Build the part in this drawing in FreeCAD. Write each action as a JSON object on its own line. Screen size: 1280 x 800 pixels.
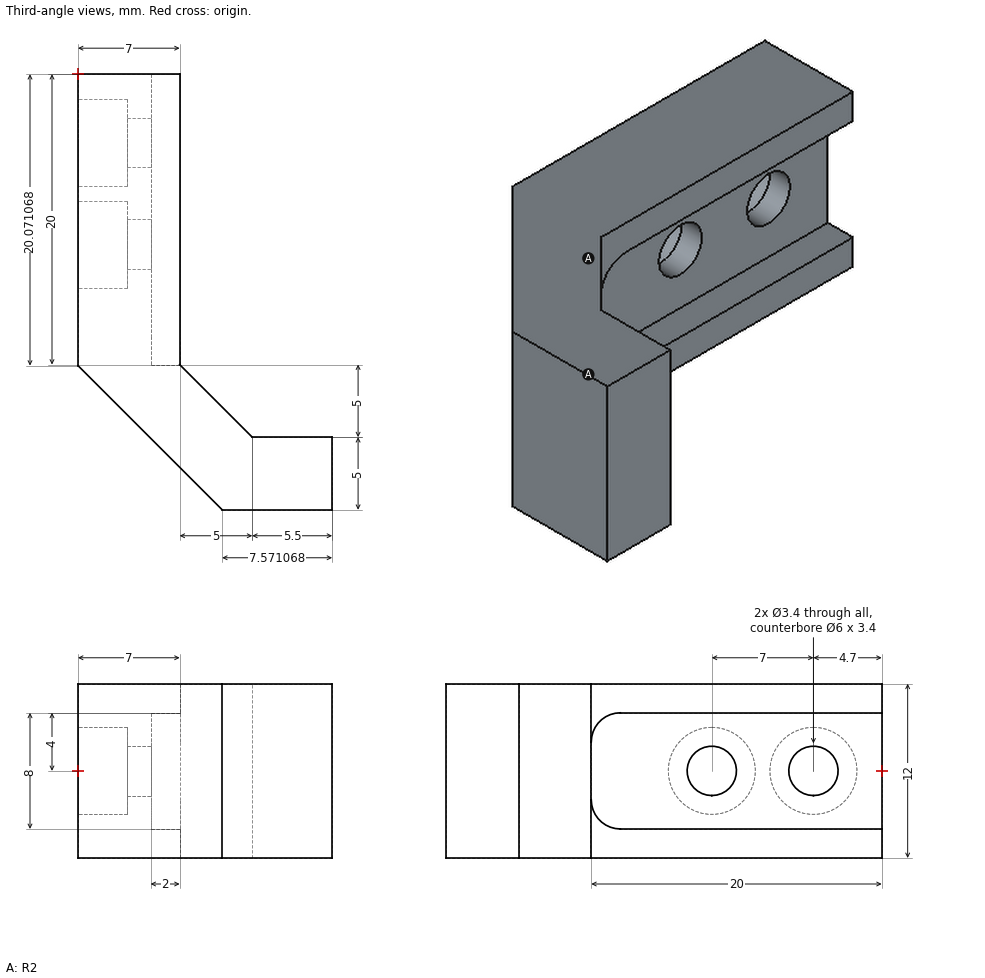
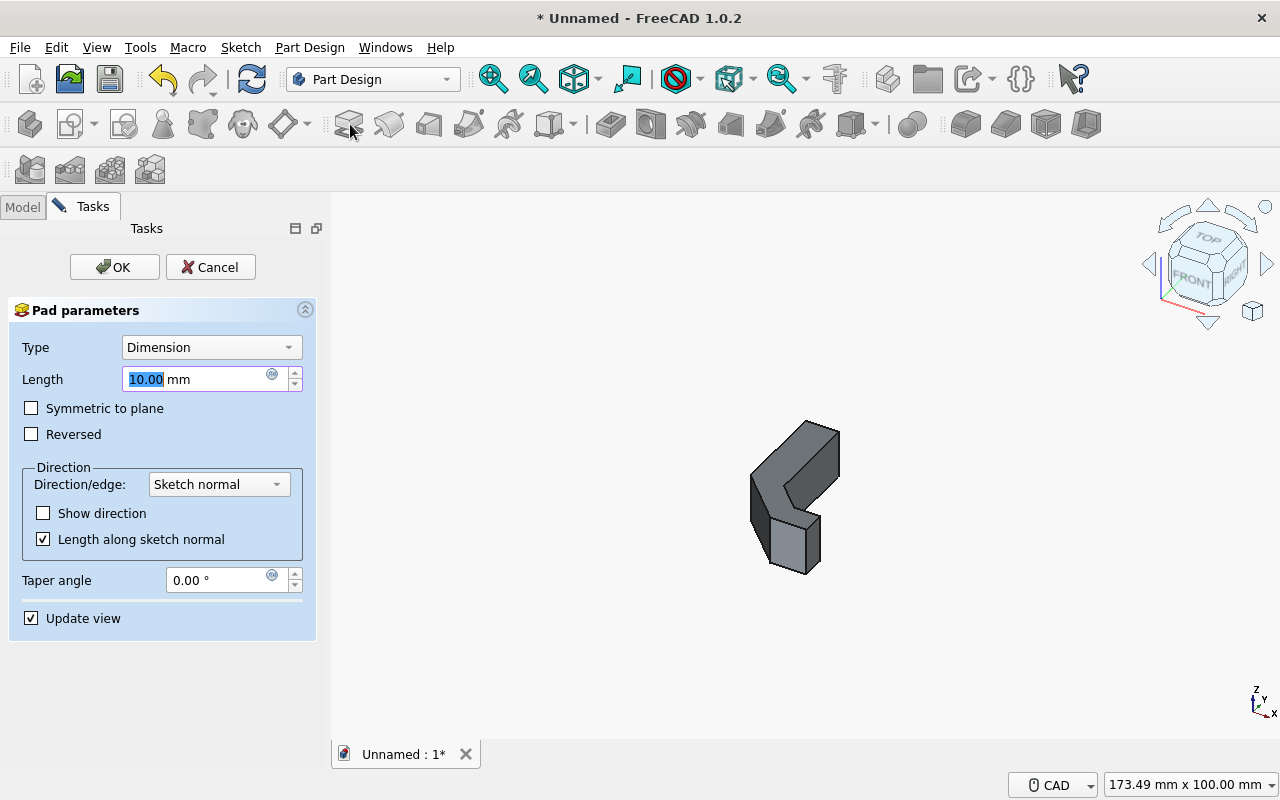
{"action": "type", "text": "12"}
{"action": "key", "text": "Tab"}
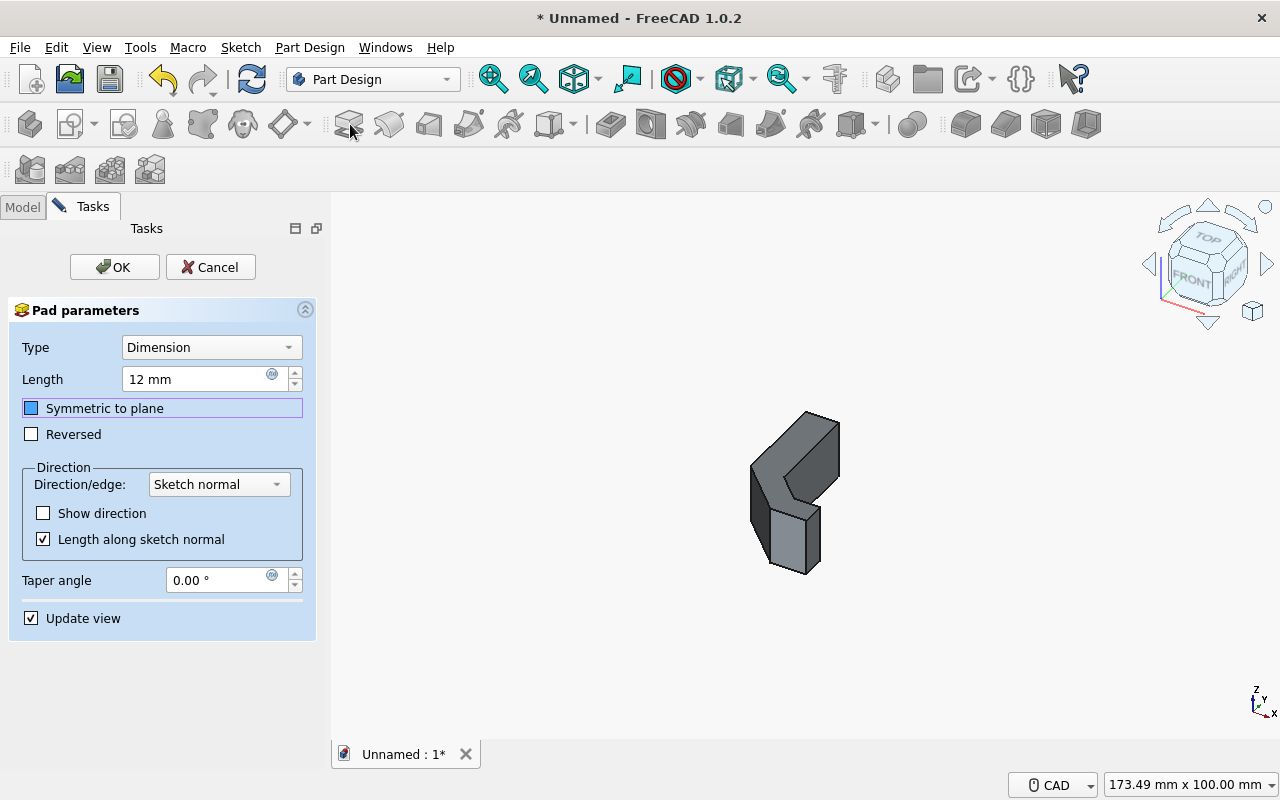
{"action": "left_click", "coordinate": [30, 408]}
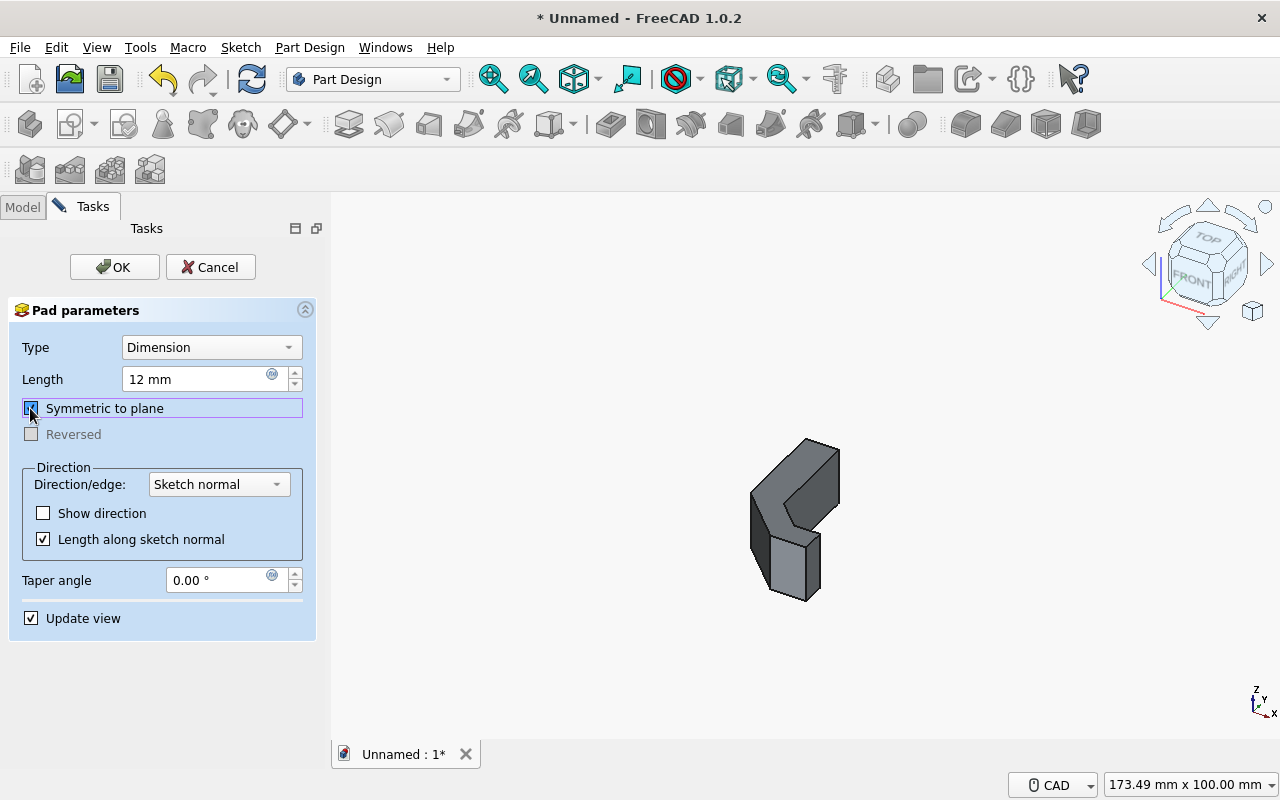
{"action": "left_click", "coordinate": [115, 267]}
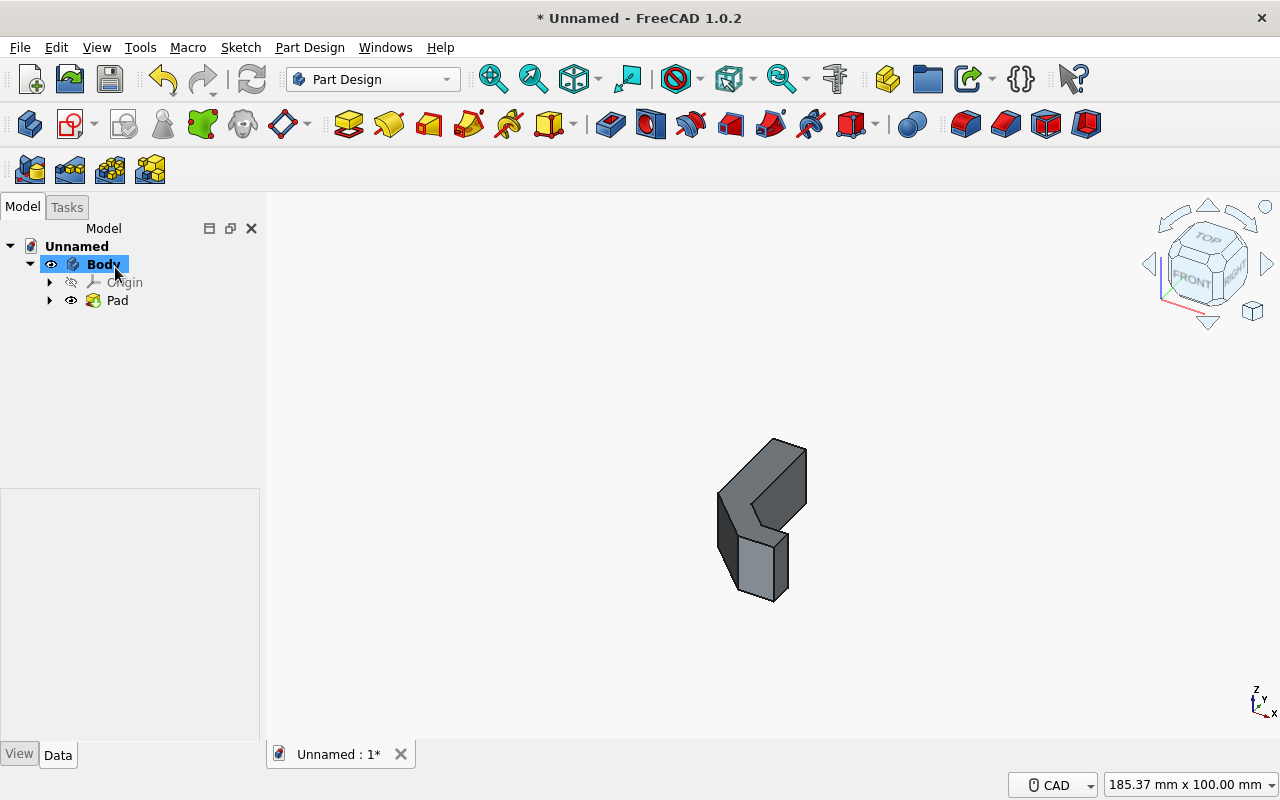
{"action": "left_click", "coordinate": [494, 80]}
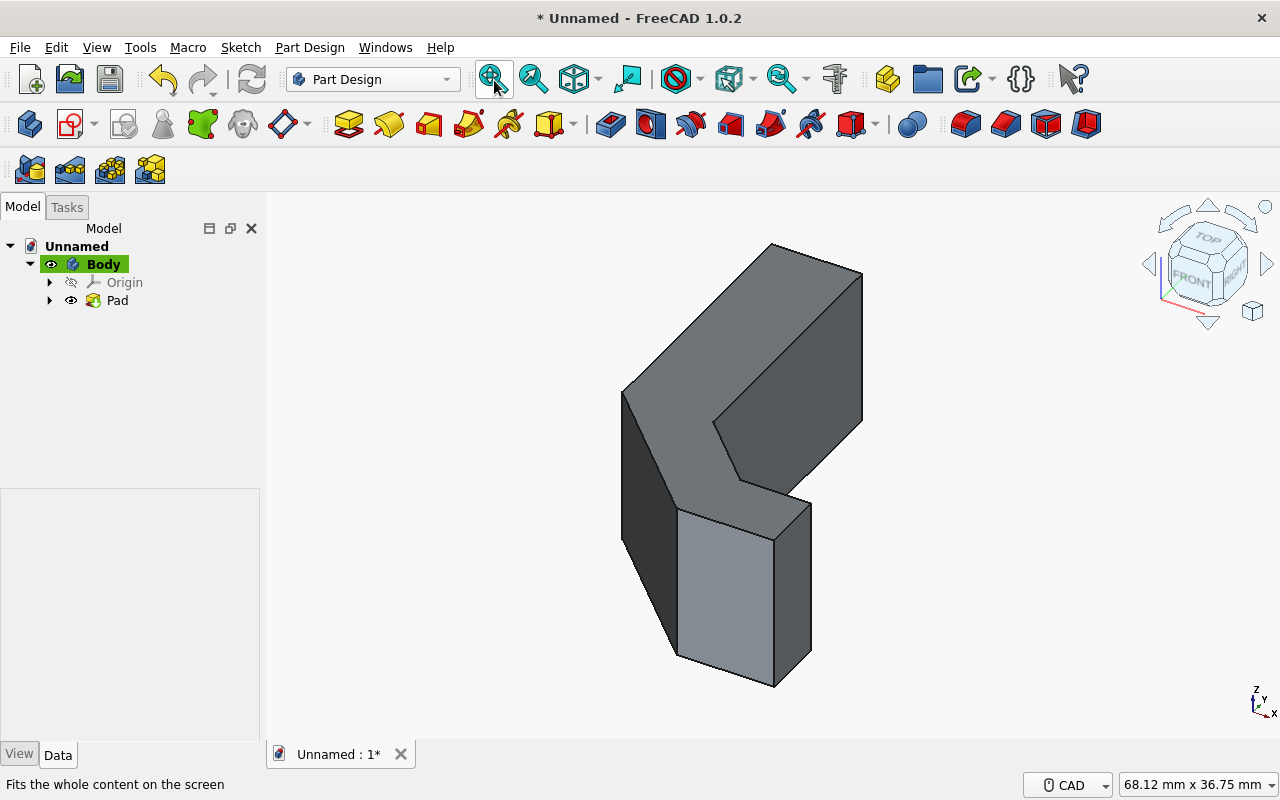
{"action": "key", "text": "4"}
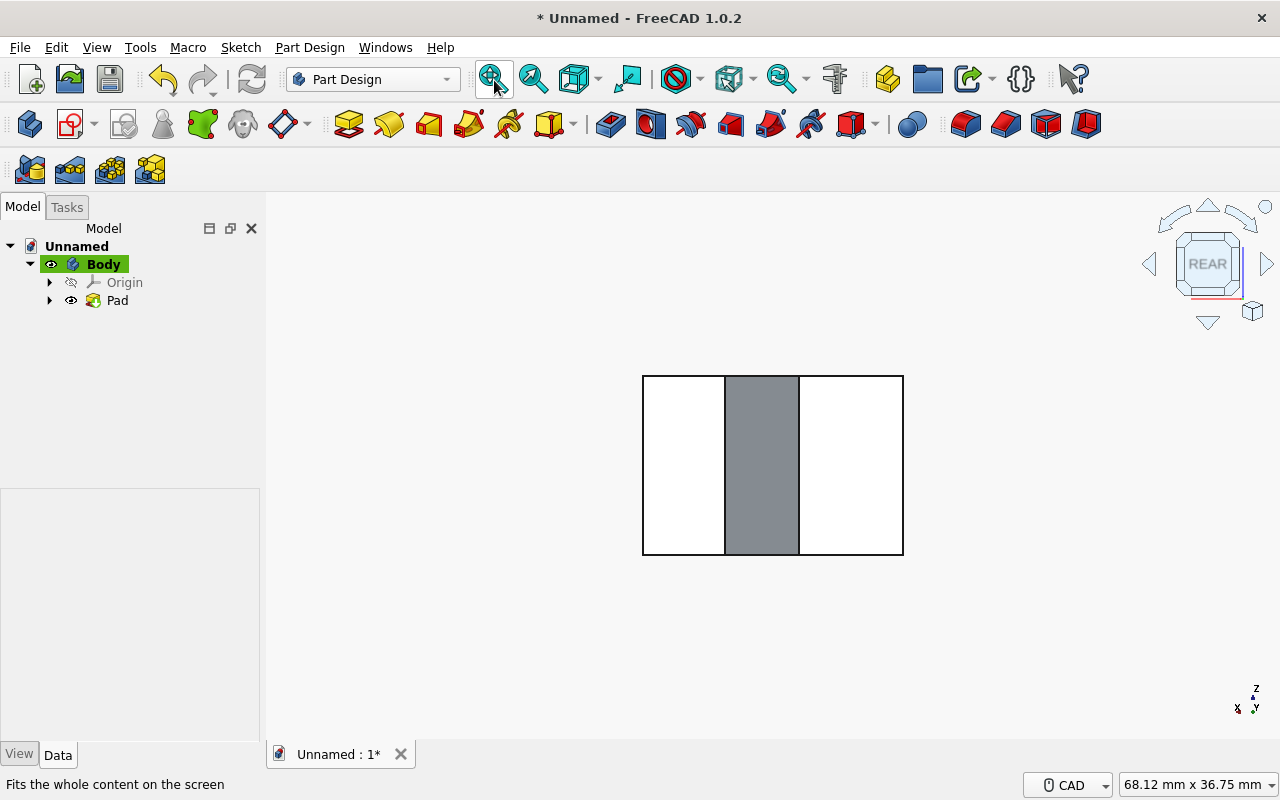
{"action": "left_click", "coordinate": [494, 80]}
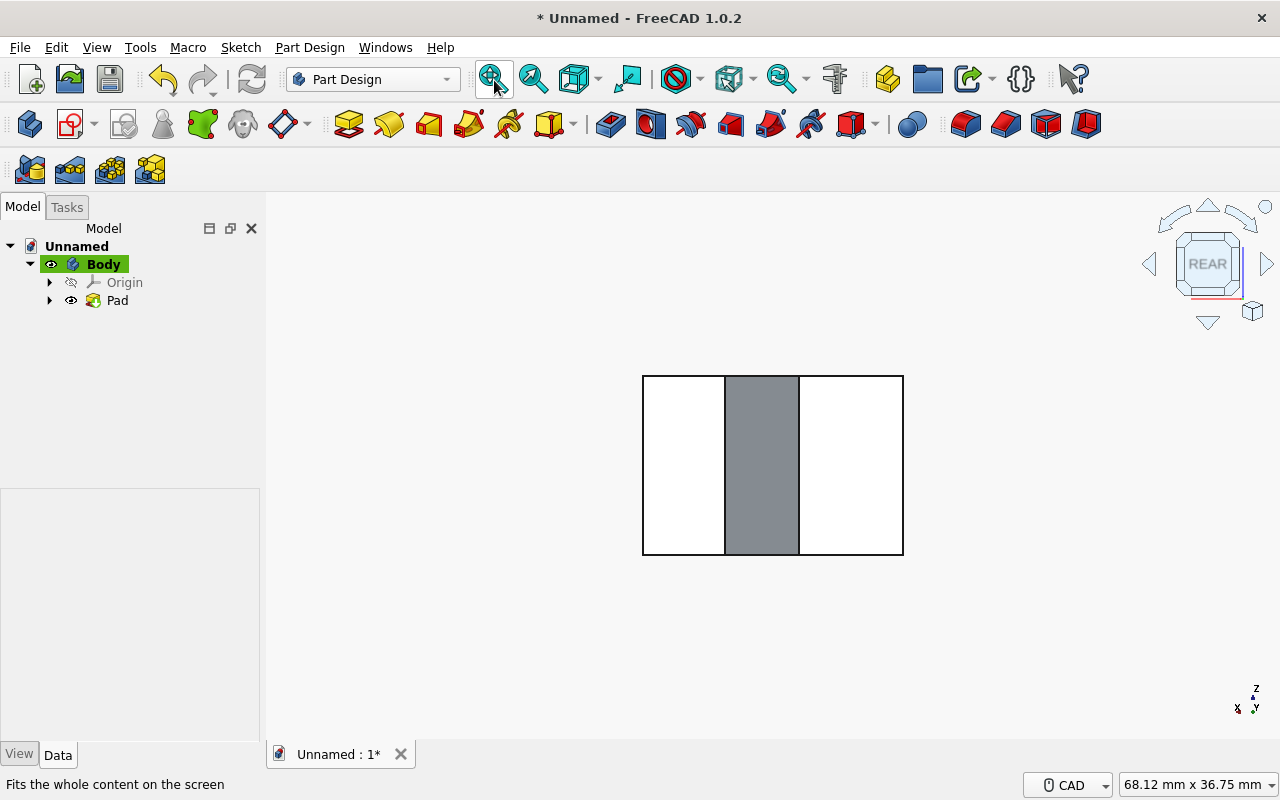
{"action": "left_click", "coordinate": [851, 439]}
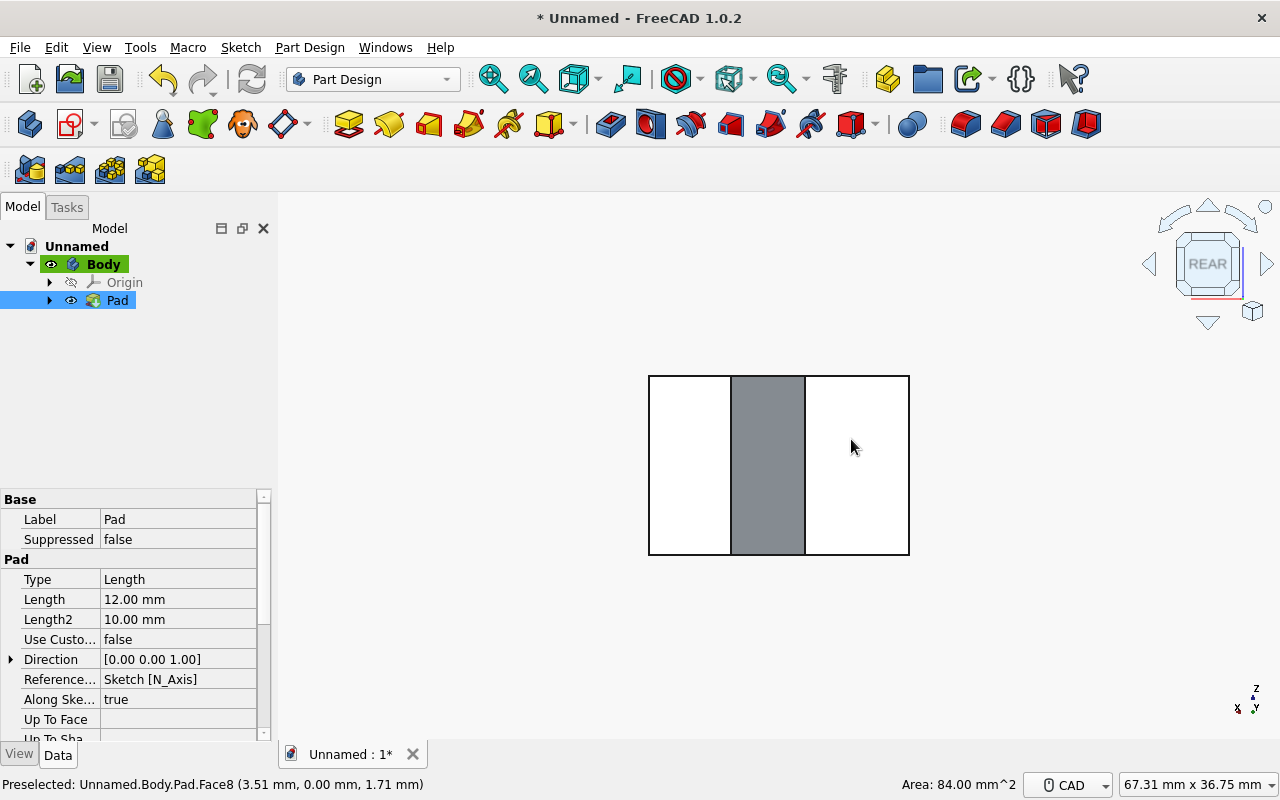
{"action": "left_click", "coordinate": [70, 124]}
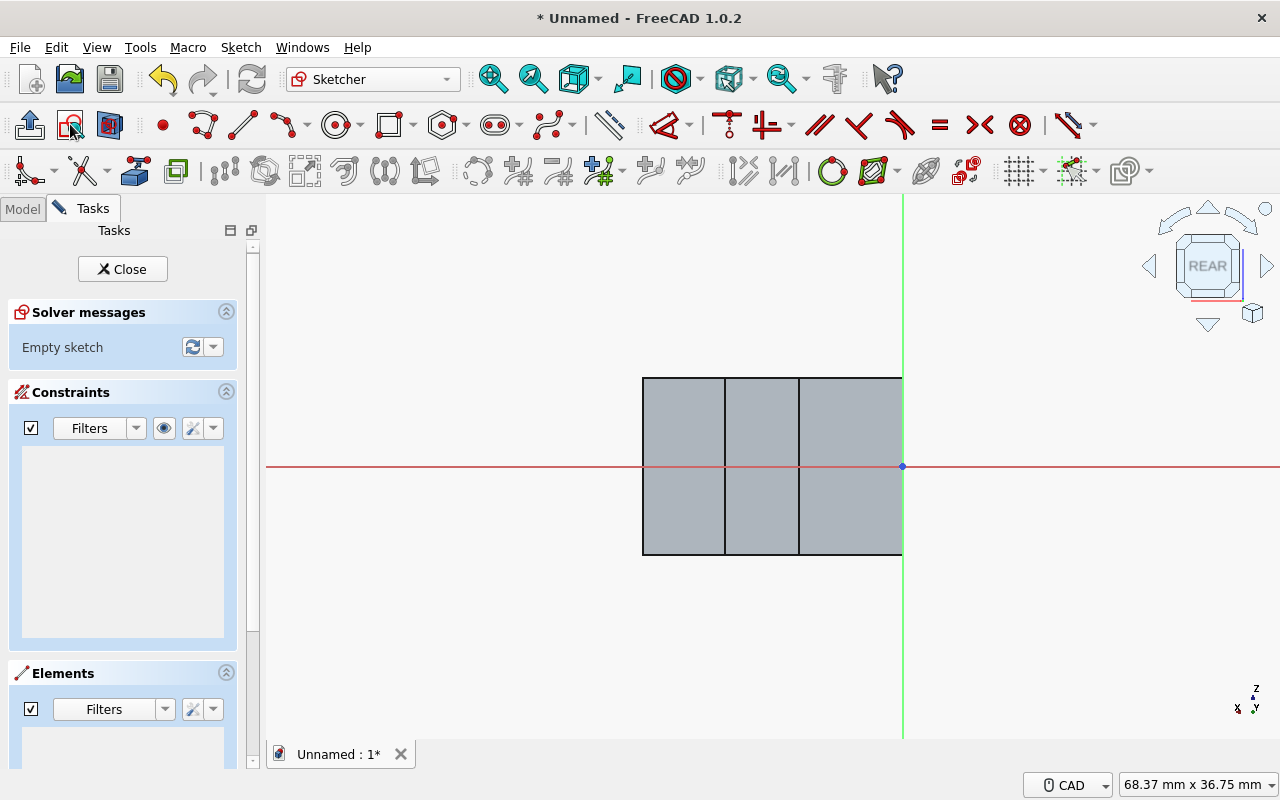
{"action": "scroll", "coordinate": [936, 466], "scroll_direction": "up", "scroll_amount": 5}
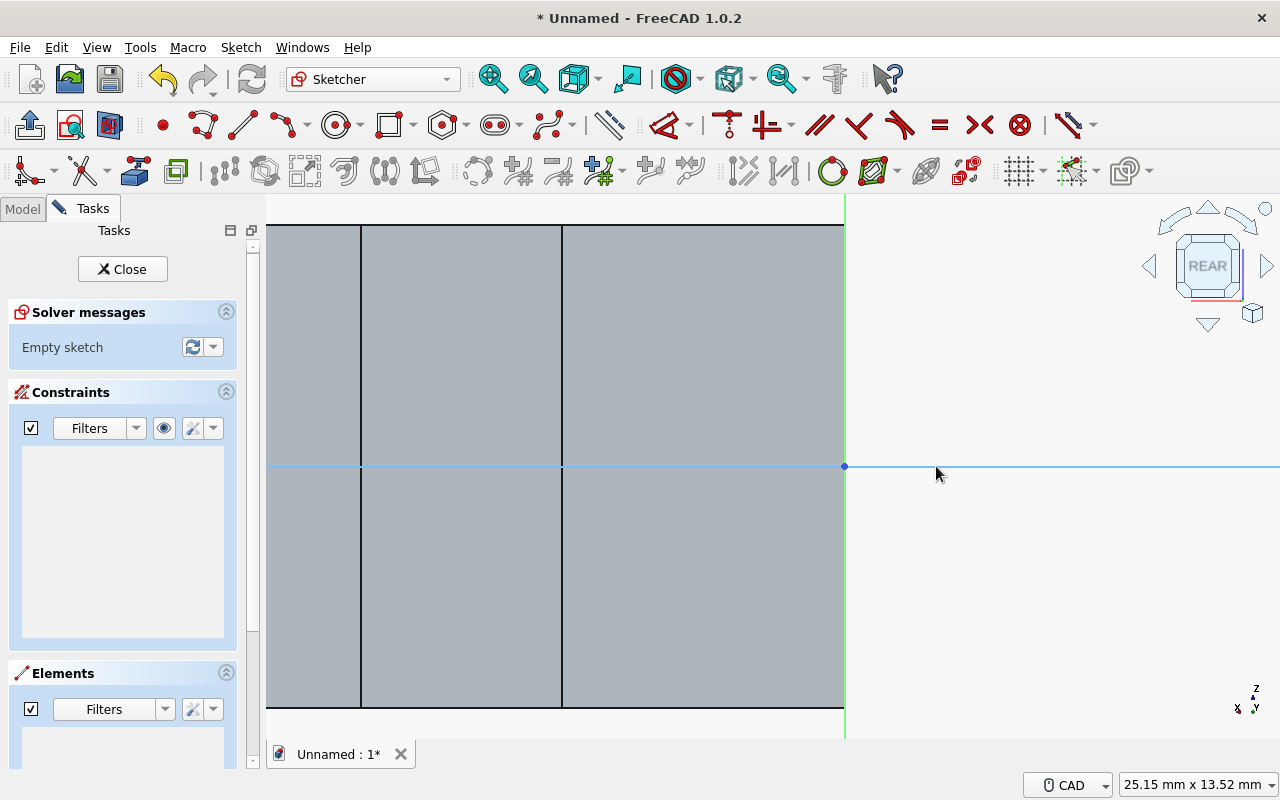
{"action": "left_click", "coordinate": [390, 126]}